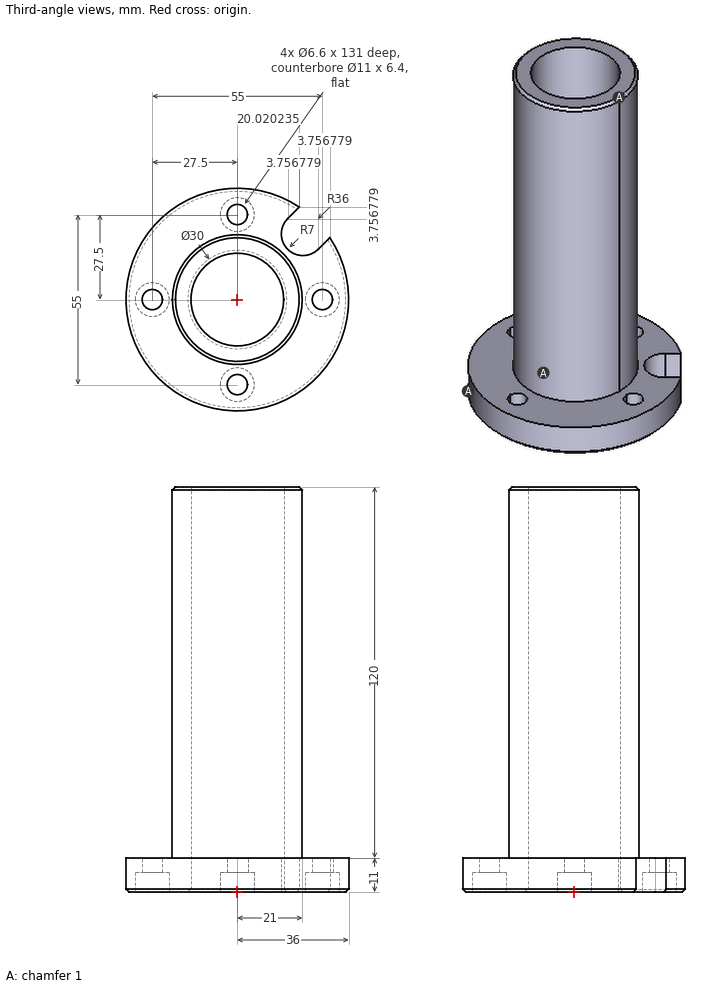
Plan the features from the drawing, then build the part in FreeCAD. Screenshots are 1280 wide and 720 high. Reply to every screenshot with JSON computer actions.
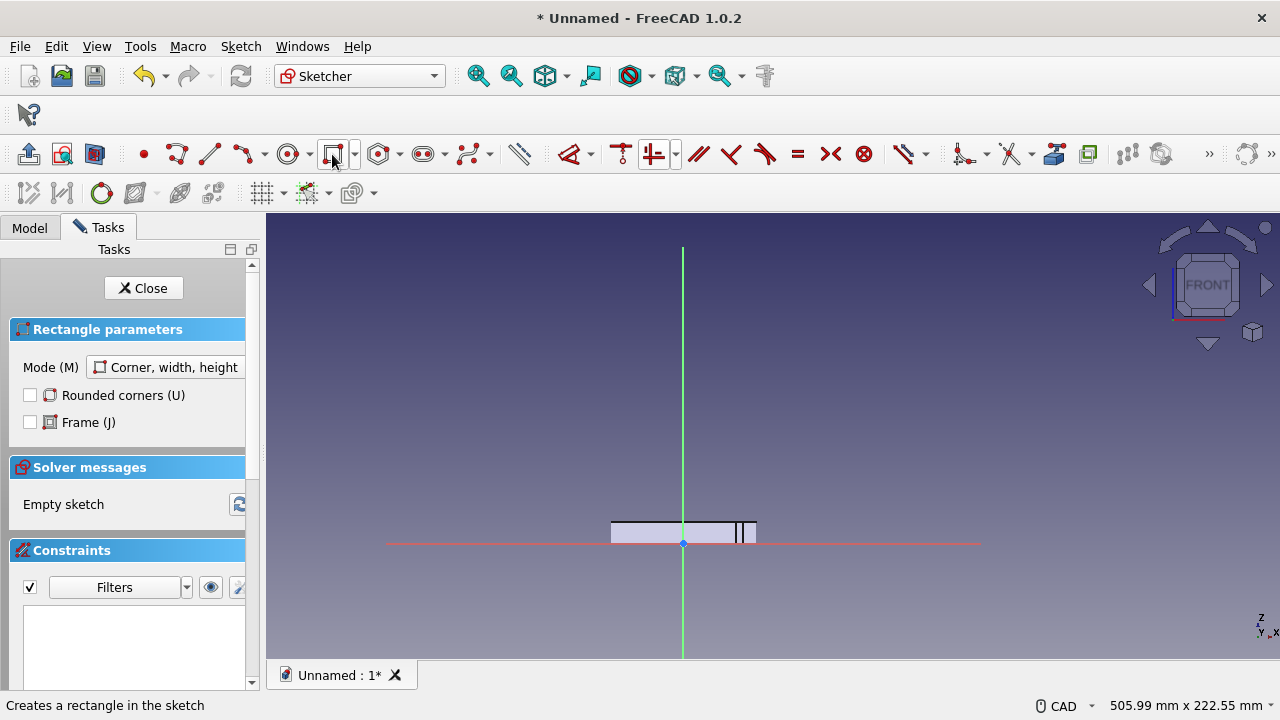
{"action": "left_click", "coordinate": [683, 281]}
{"action": "mouse_move", "coordinate": [726, 522]}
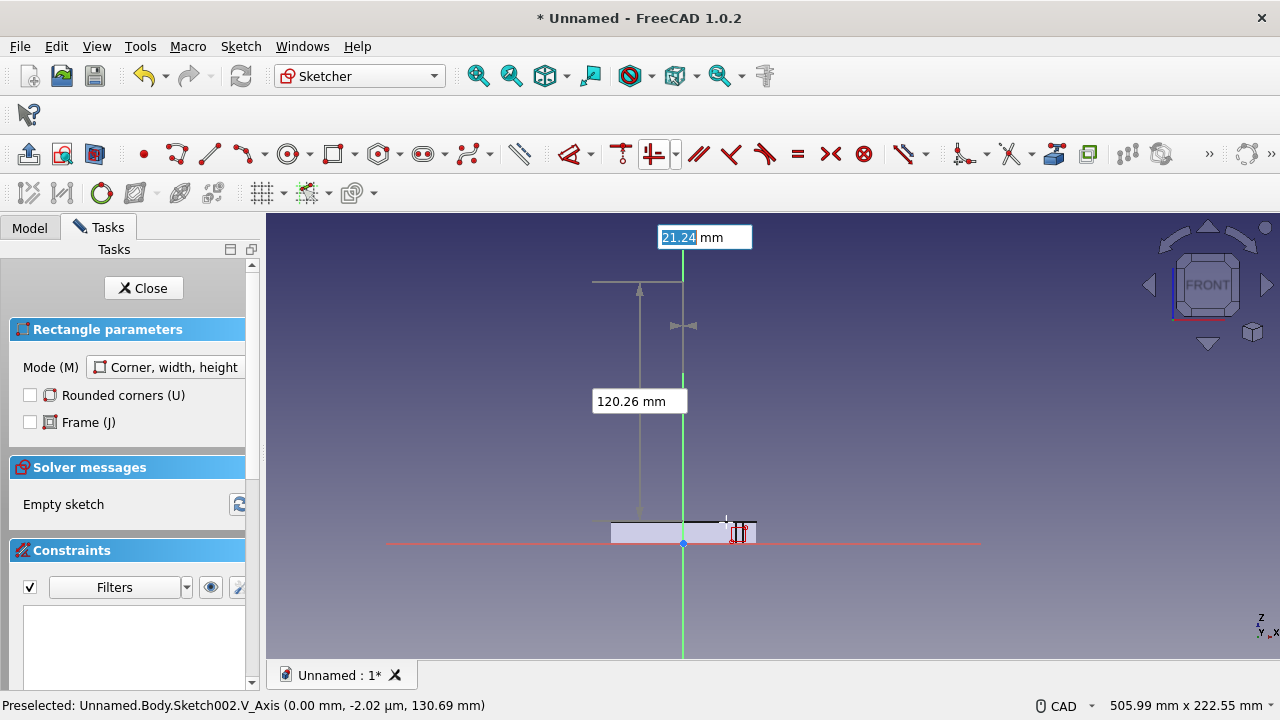
{"action": "type", "text": "21"}
{"action": "key", "text": "Tab"}
{"action": "type", "text": "120"}
{"action": "key", "text": "Return"}
{"action": "key", "text": "Escape"}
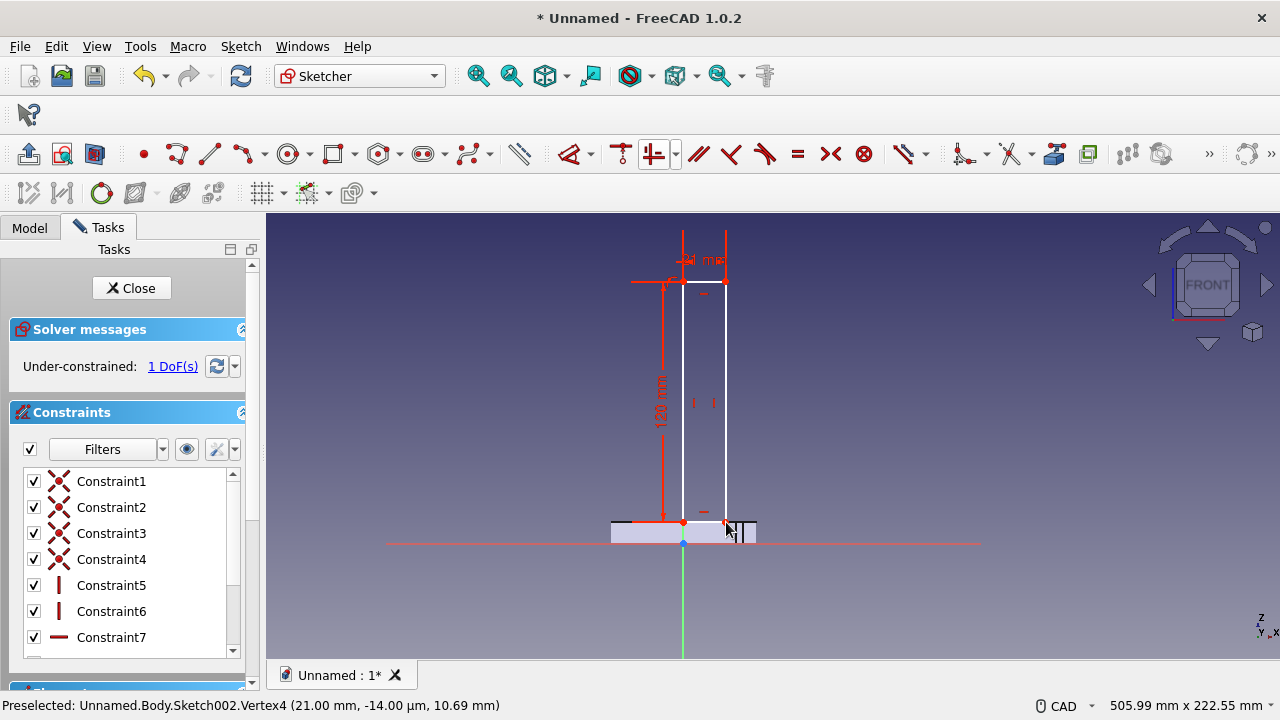
{"action": "key", "text": "d"}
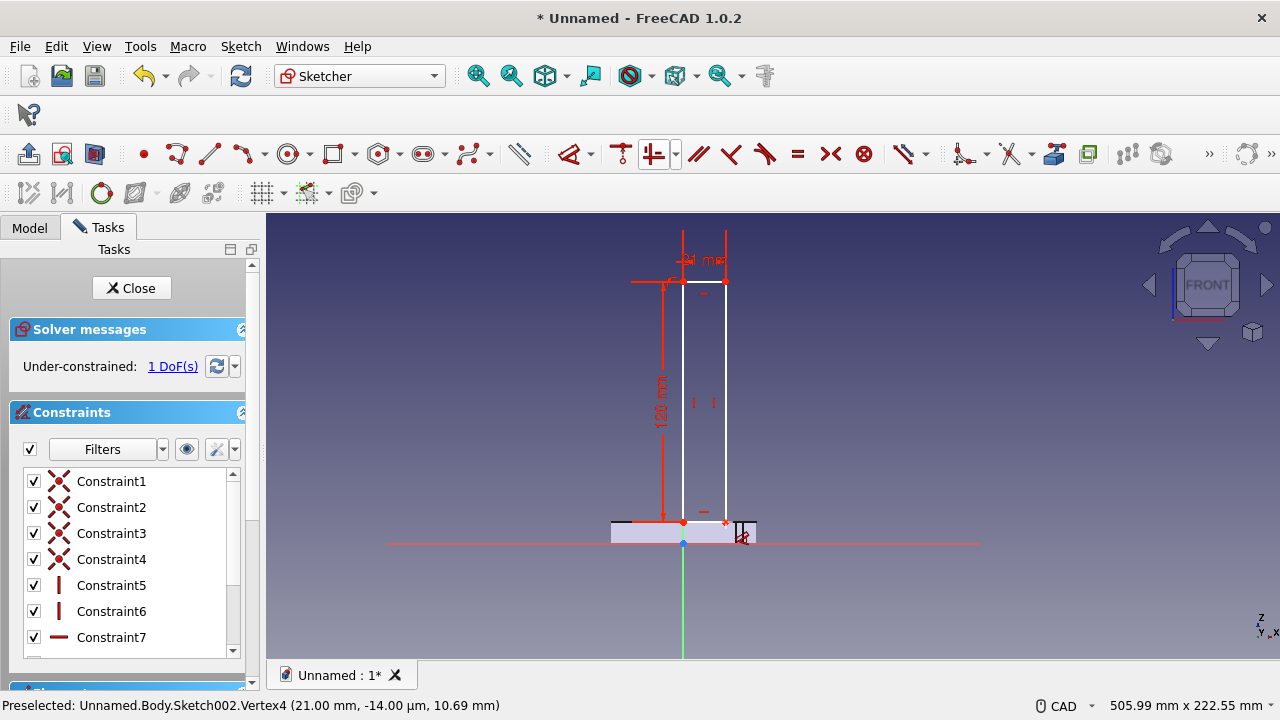
{"action": "scroll", "coordinate": [683, 522], "scroll_direction": "up", "scroll_amount": 3}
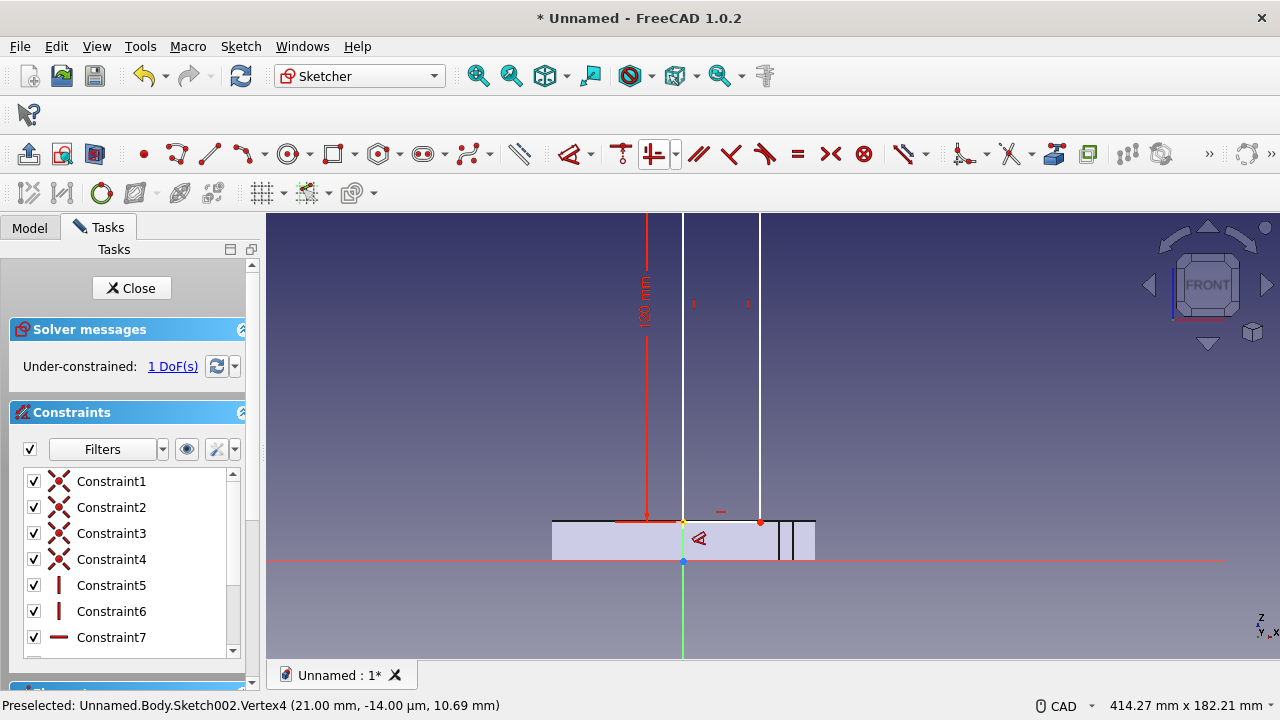
{"action": "left_click", "coordinate": [683, 522]}
{"action": "left_click", "coordinate": [649, 542]}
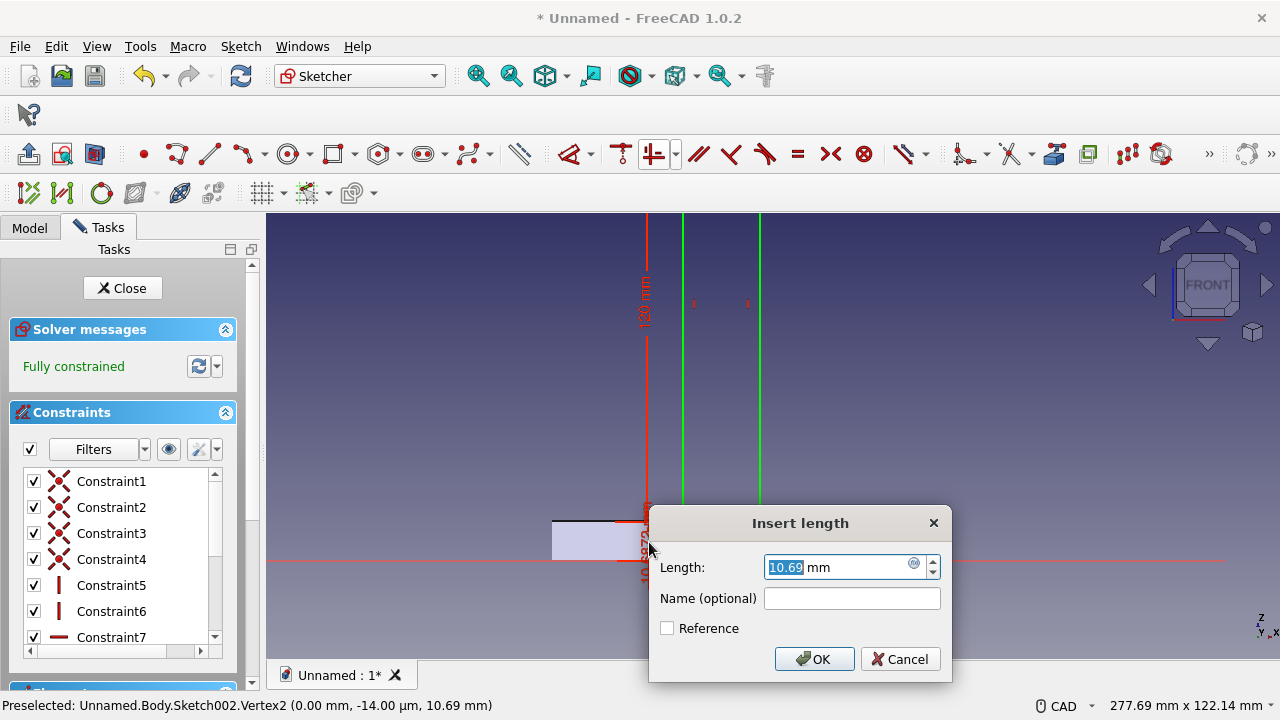
{"action": "type", "text": "11"}
{"action": "key", "text": "Return"}
{"action": "key", "text": "Escape"}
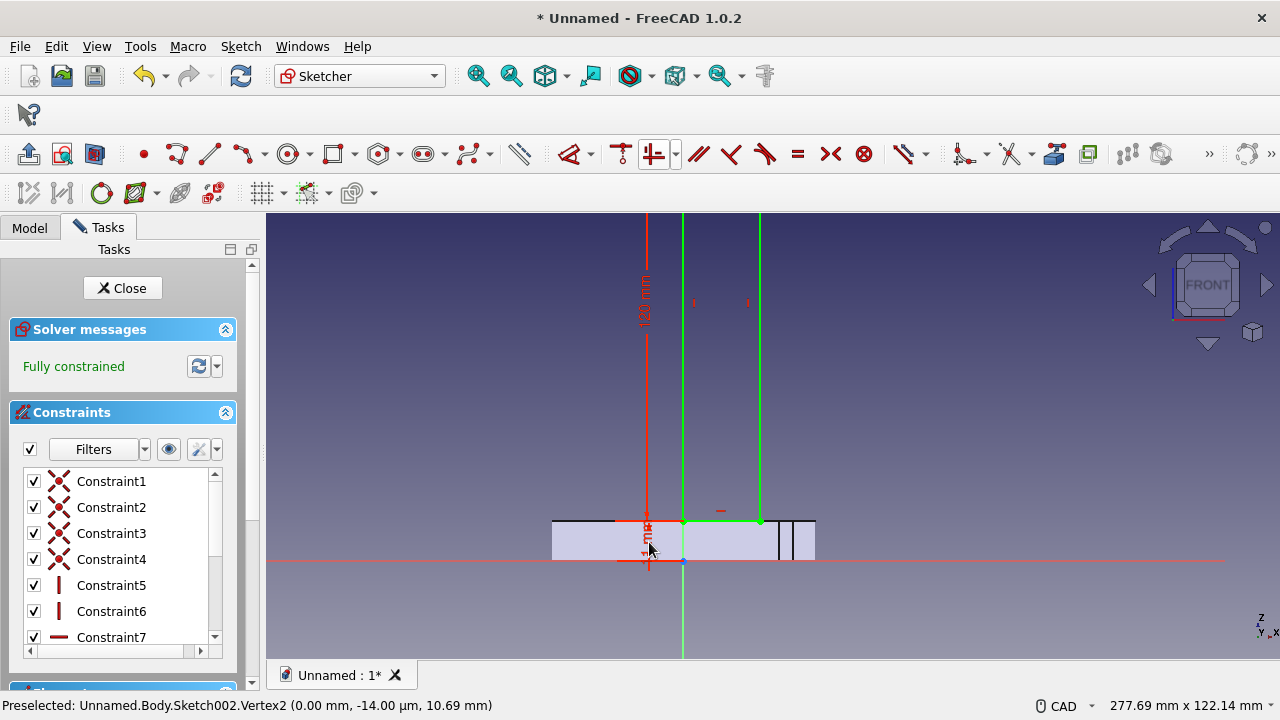
{"action": "left_click", "coordinate": [123, 288]}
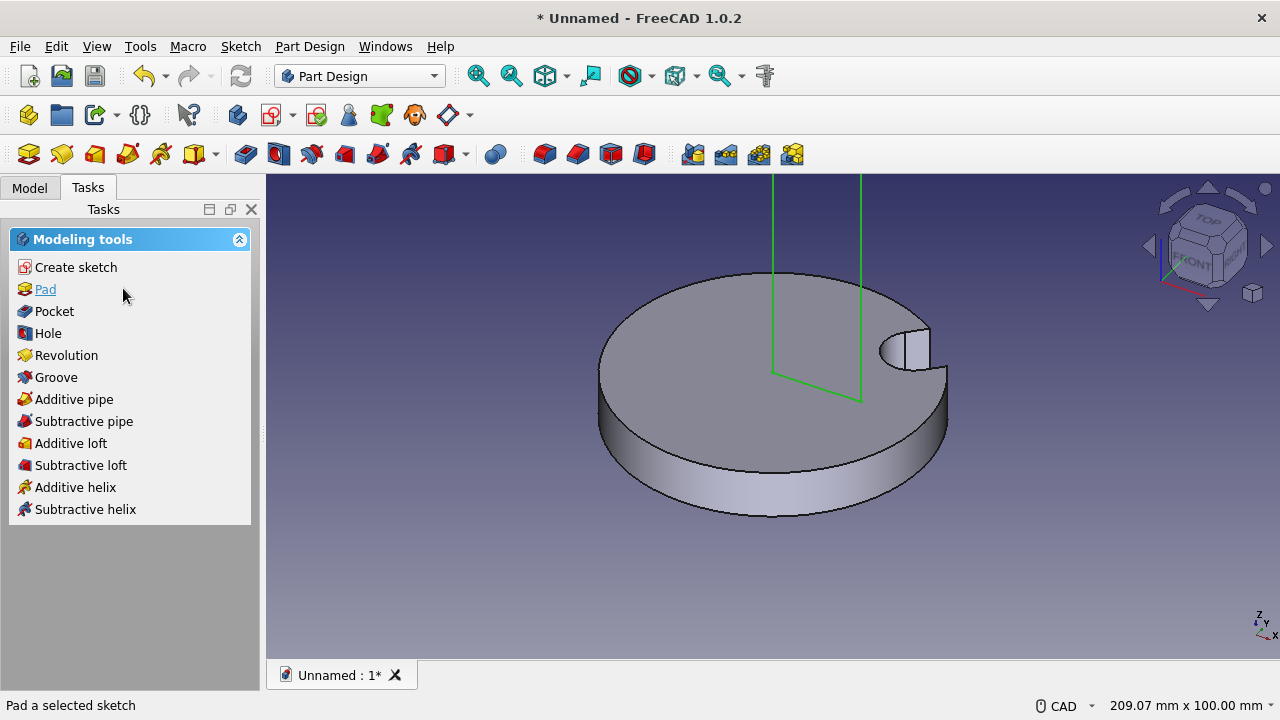
{"action": "left_click", "coordinate": [62, 154]}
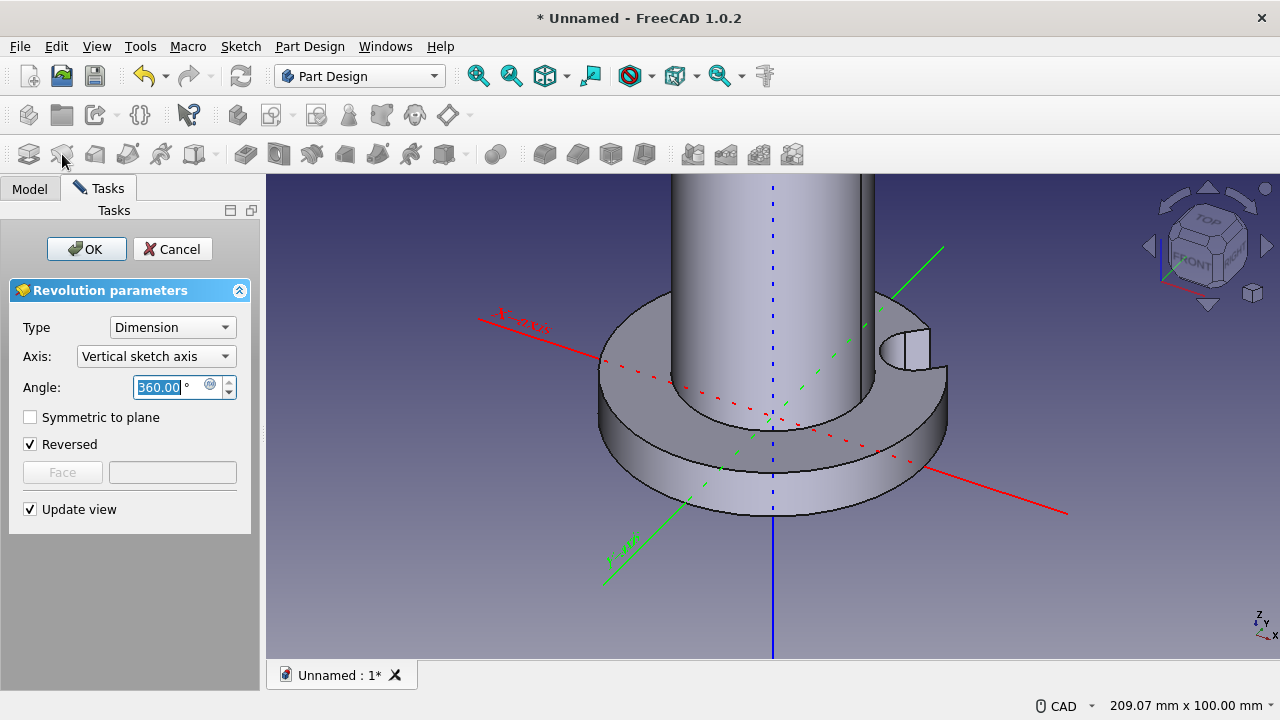
{"action": "left_click", "coordinate": [87, 249]}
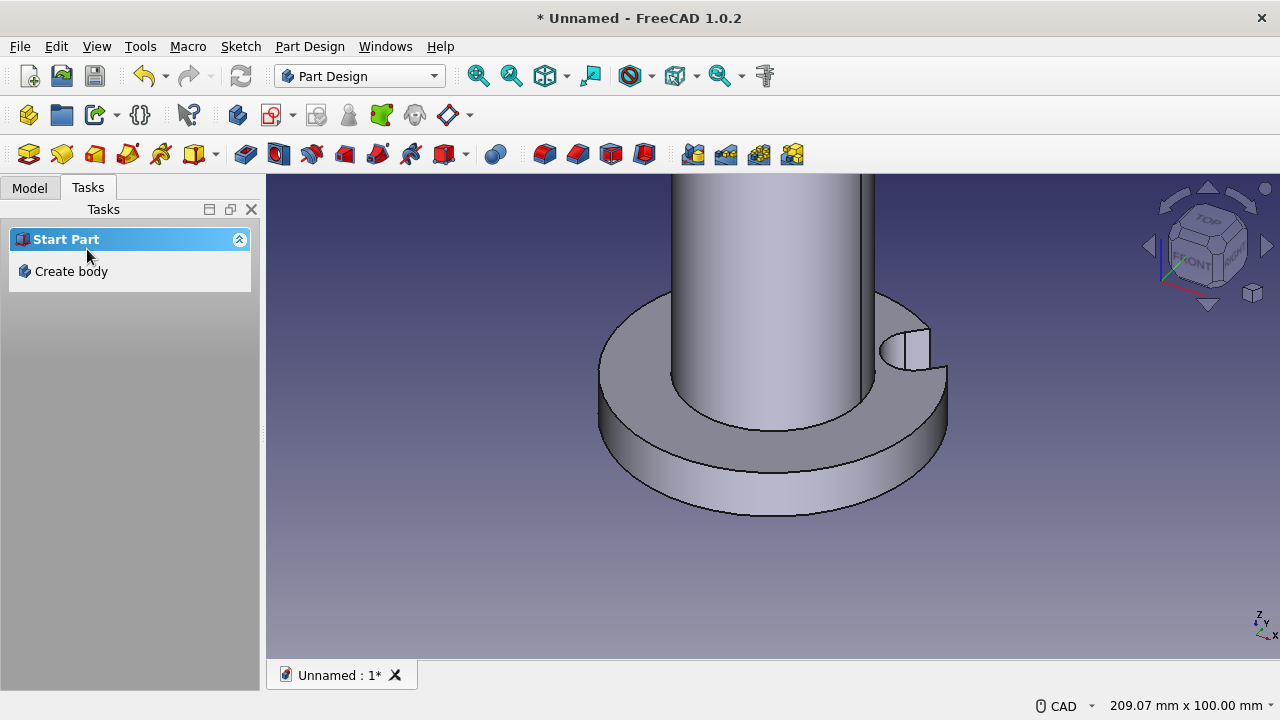
{"action": "left_click", "coordinate": [479, 76]}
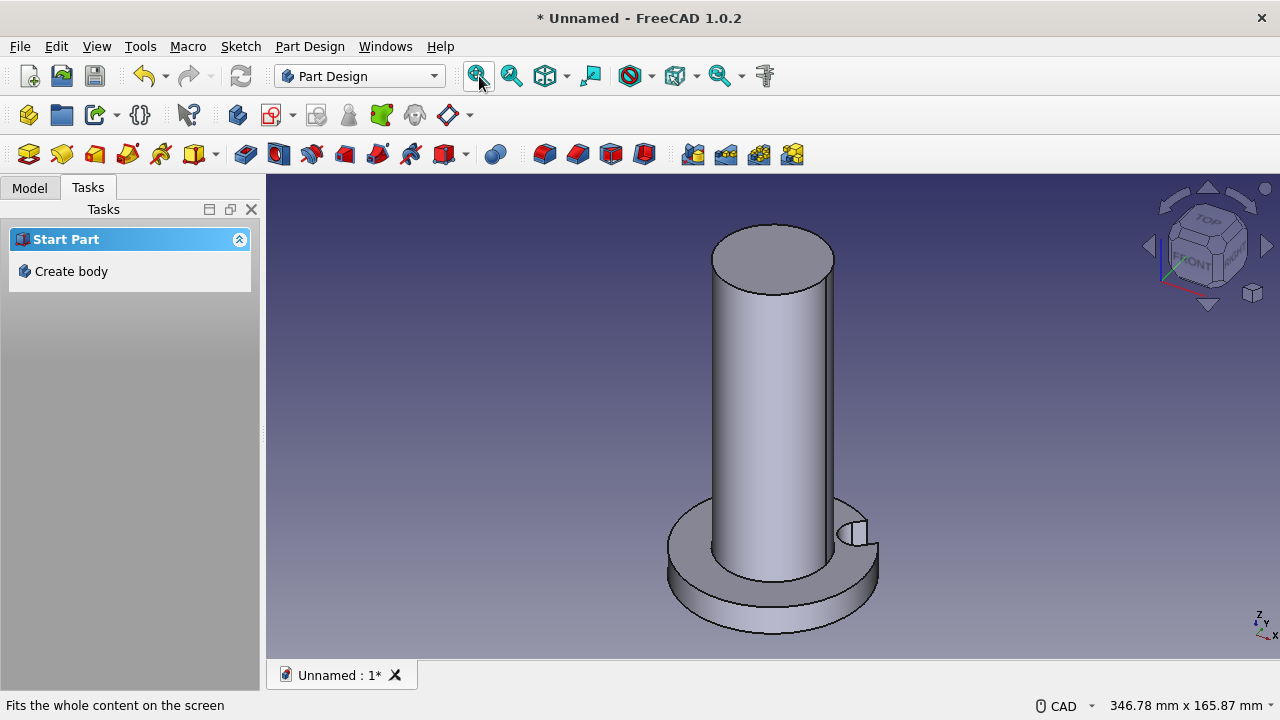
{"action": "key", "text": "5"}